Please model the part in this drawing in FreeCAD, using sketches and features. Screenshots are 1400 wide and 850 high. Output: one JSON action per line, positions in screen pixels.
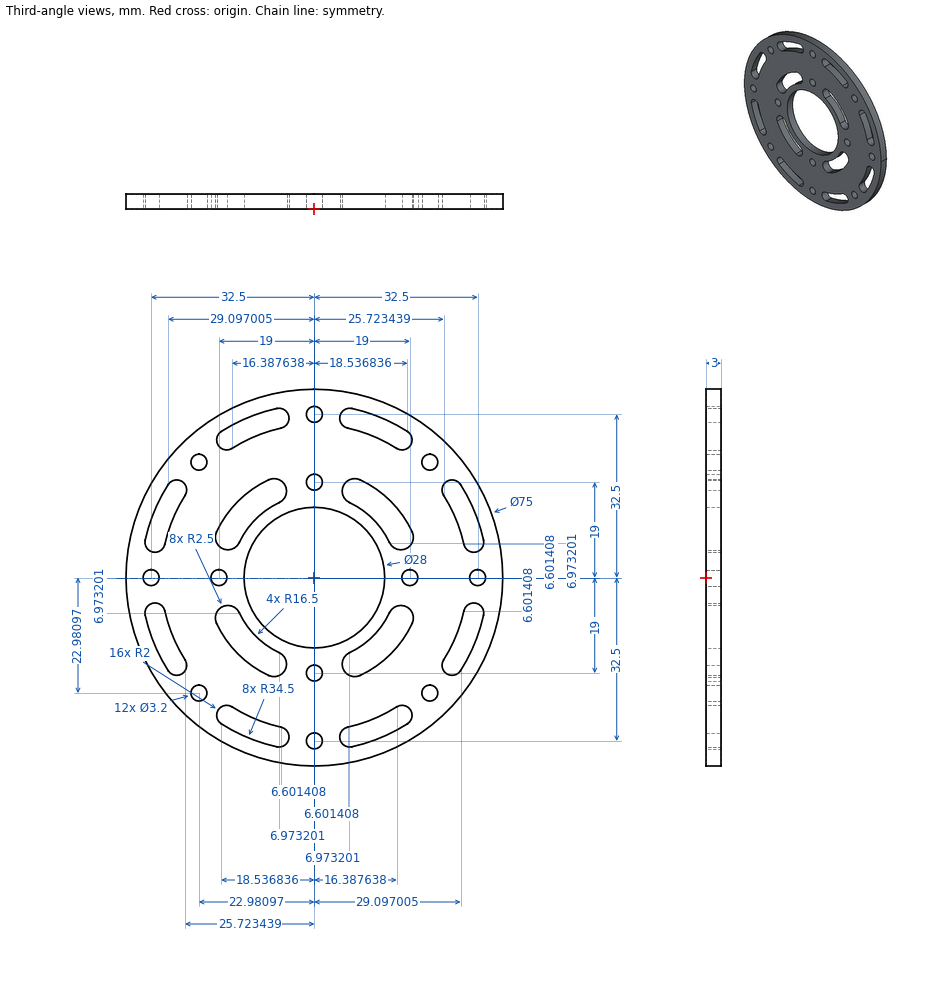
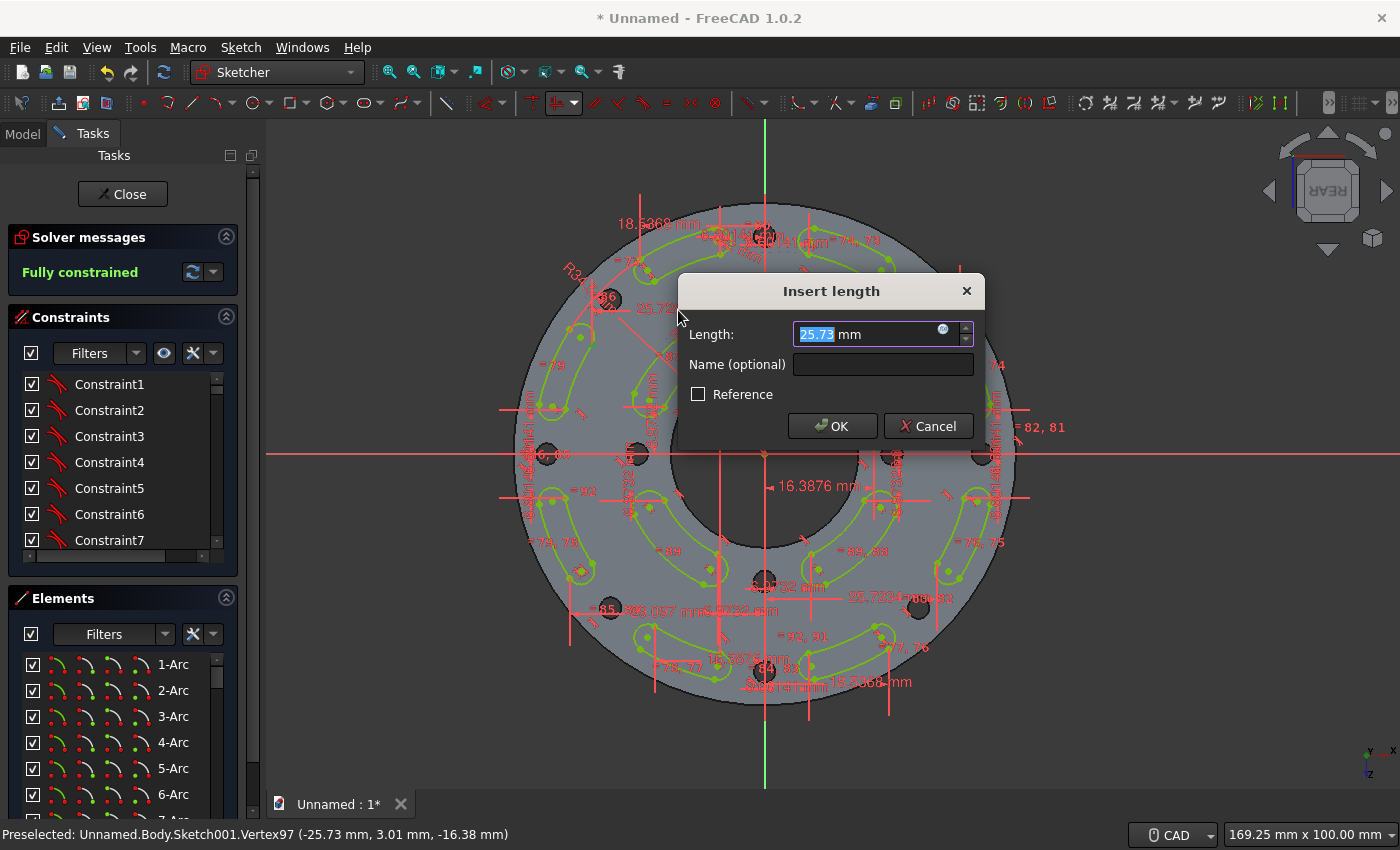
{"action": "type", "text": "25.723439"}
{"action": "key", "text": "Return"}
{"action": "key", "text": "Escape"}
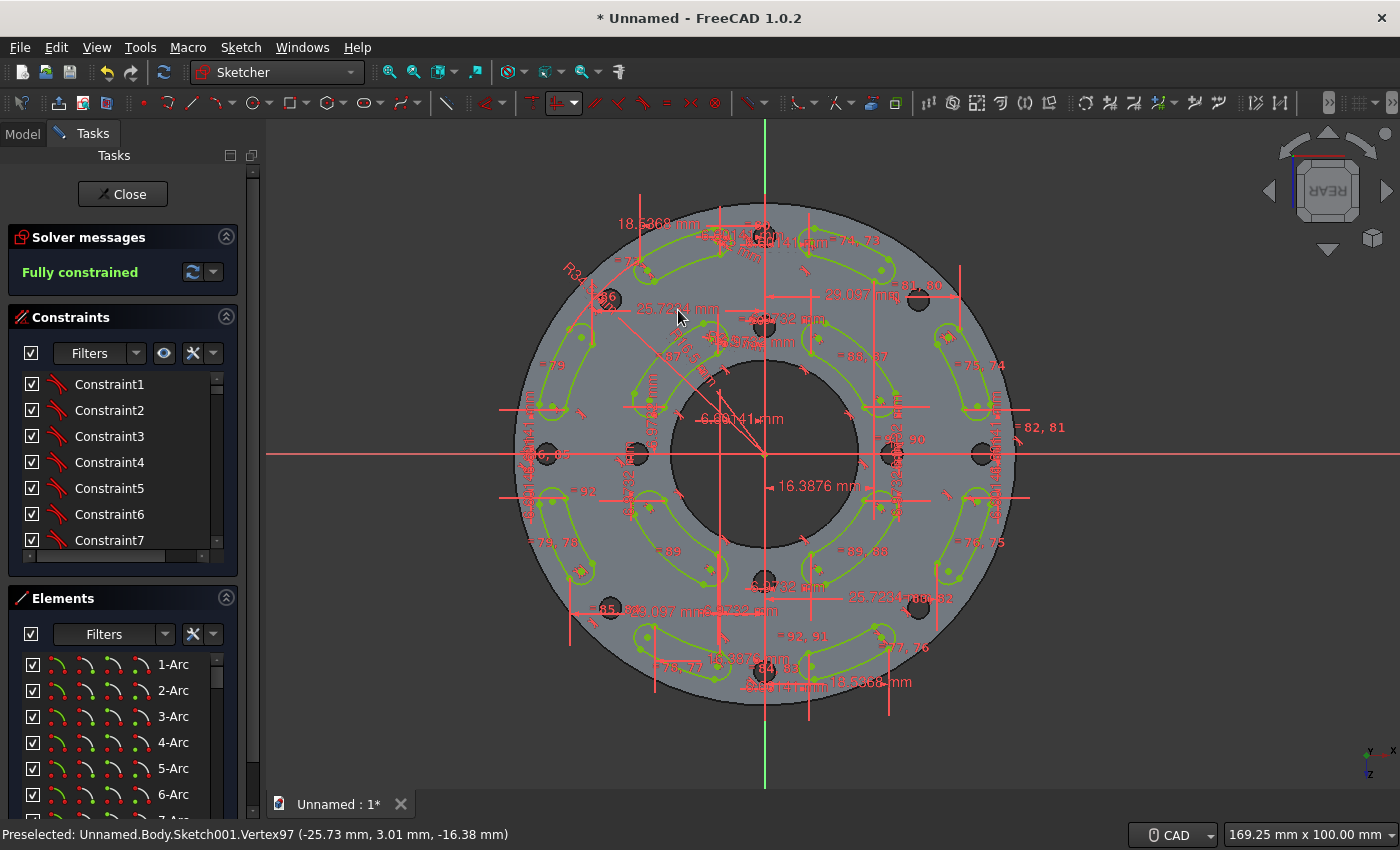
{"action": "left_click", "coordinate": [123, 194]}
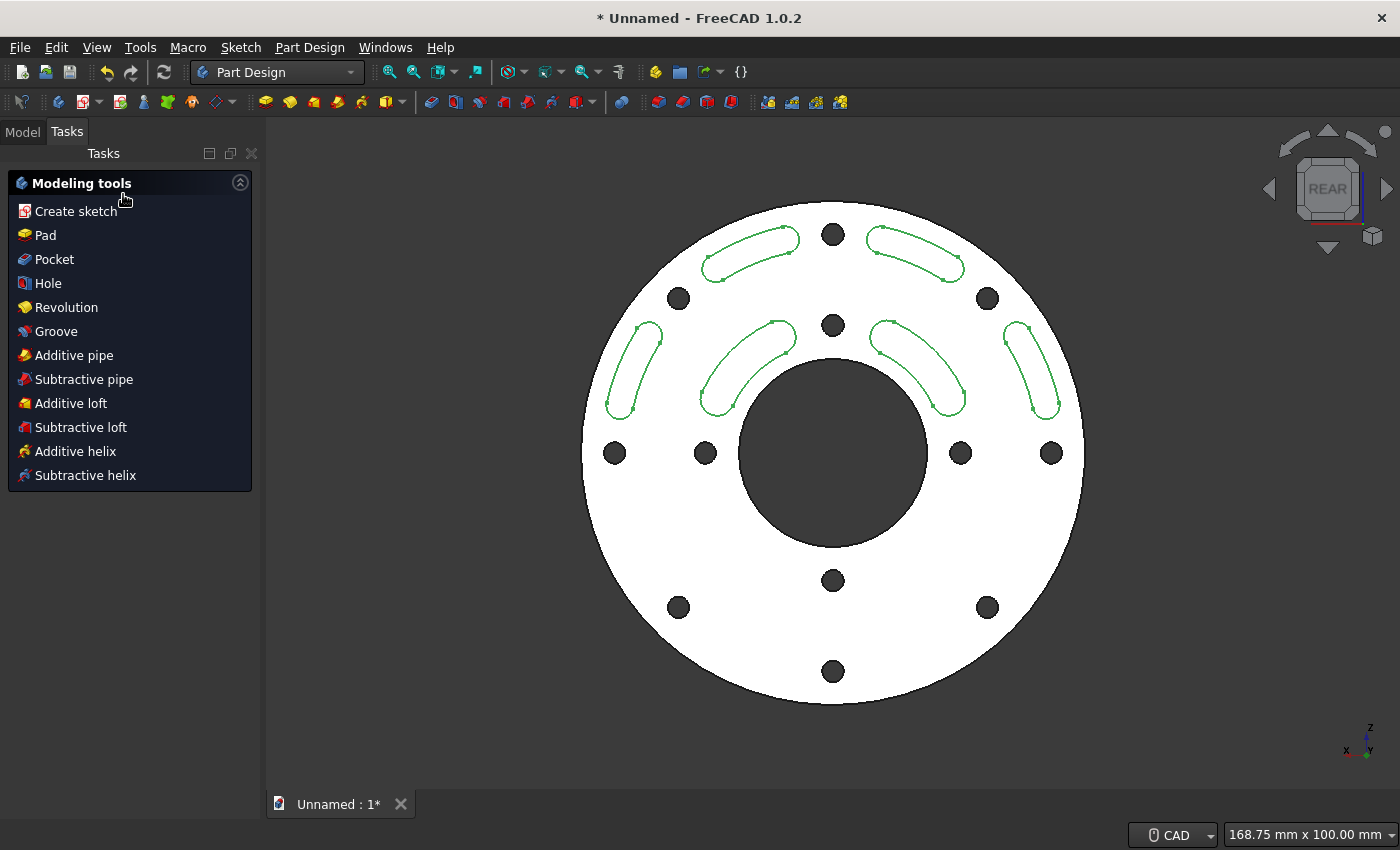
{"action": "left_click", "coordinate": [432, 102]}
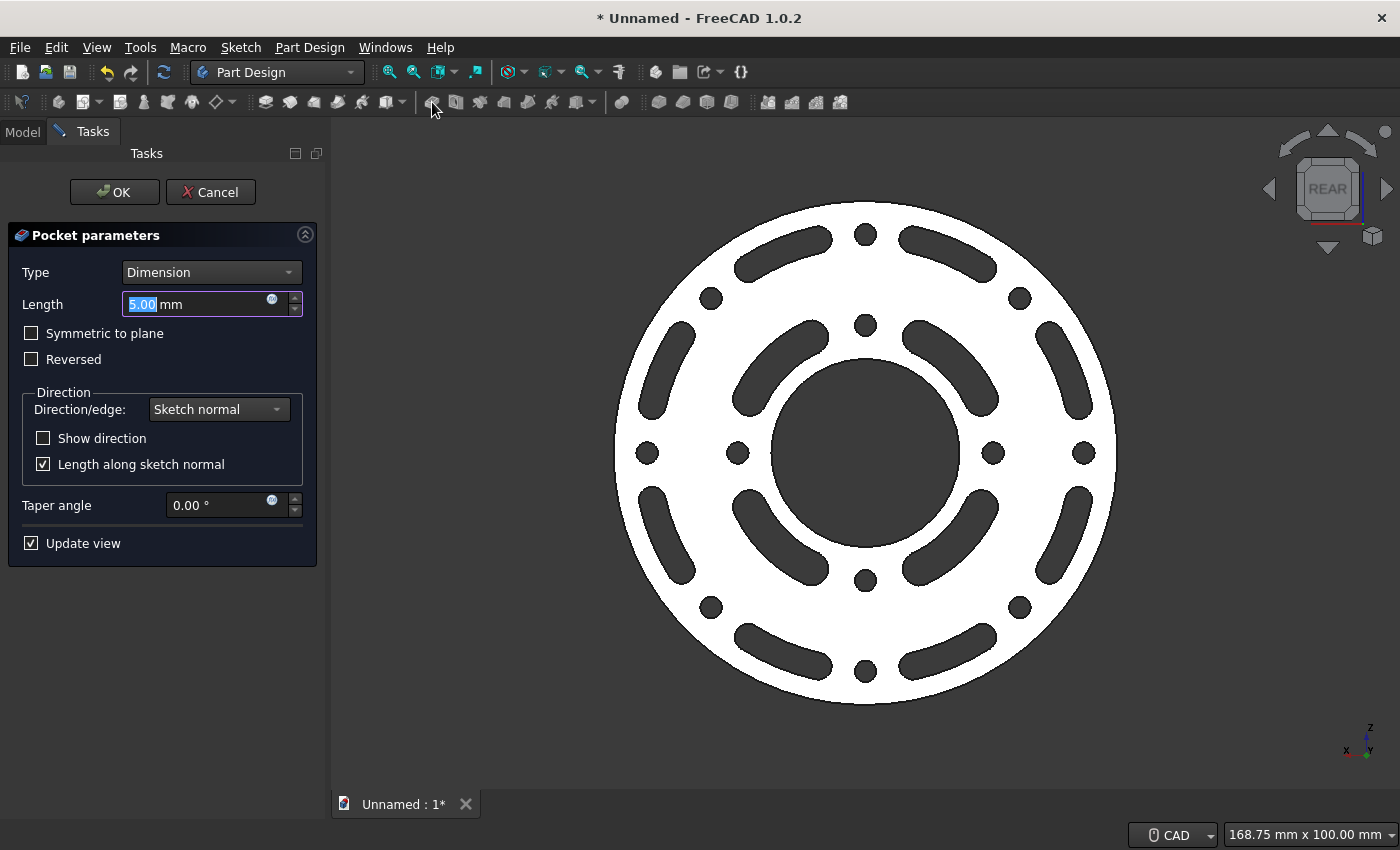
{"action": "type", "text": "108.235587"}
{"action": "key", "text": "Tab"}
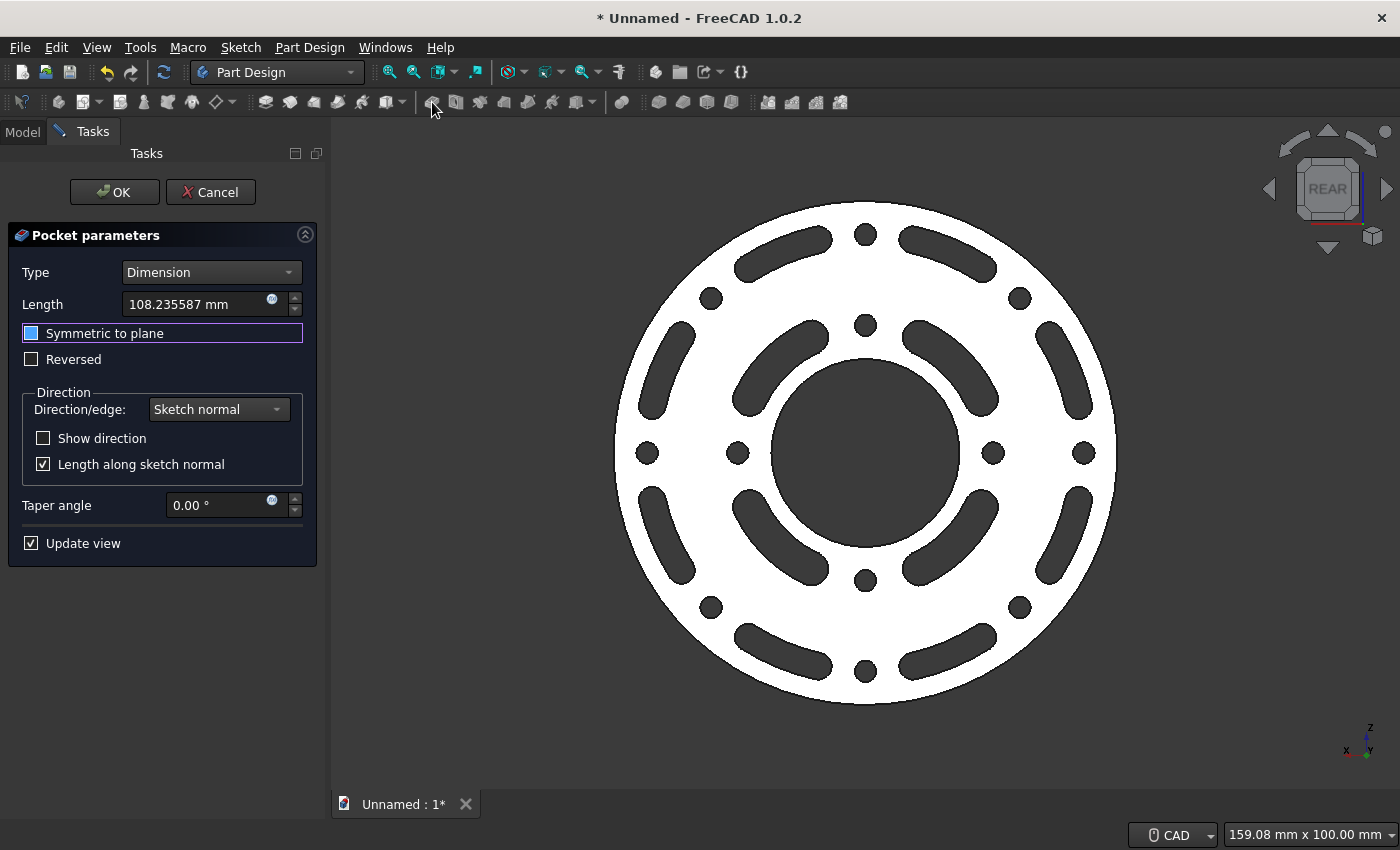
{"action": "left_click", "coordinate": [30, 333]}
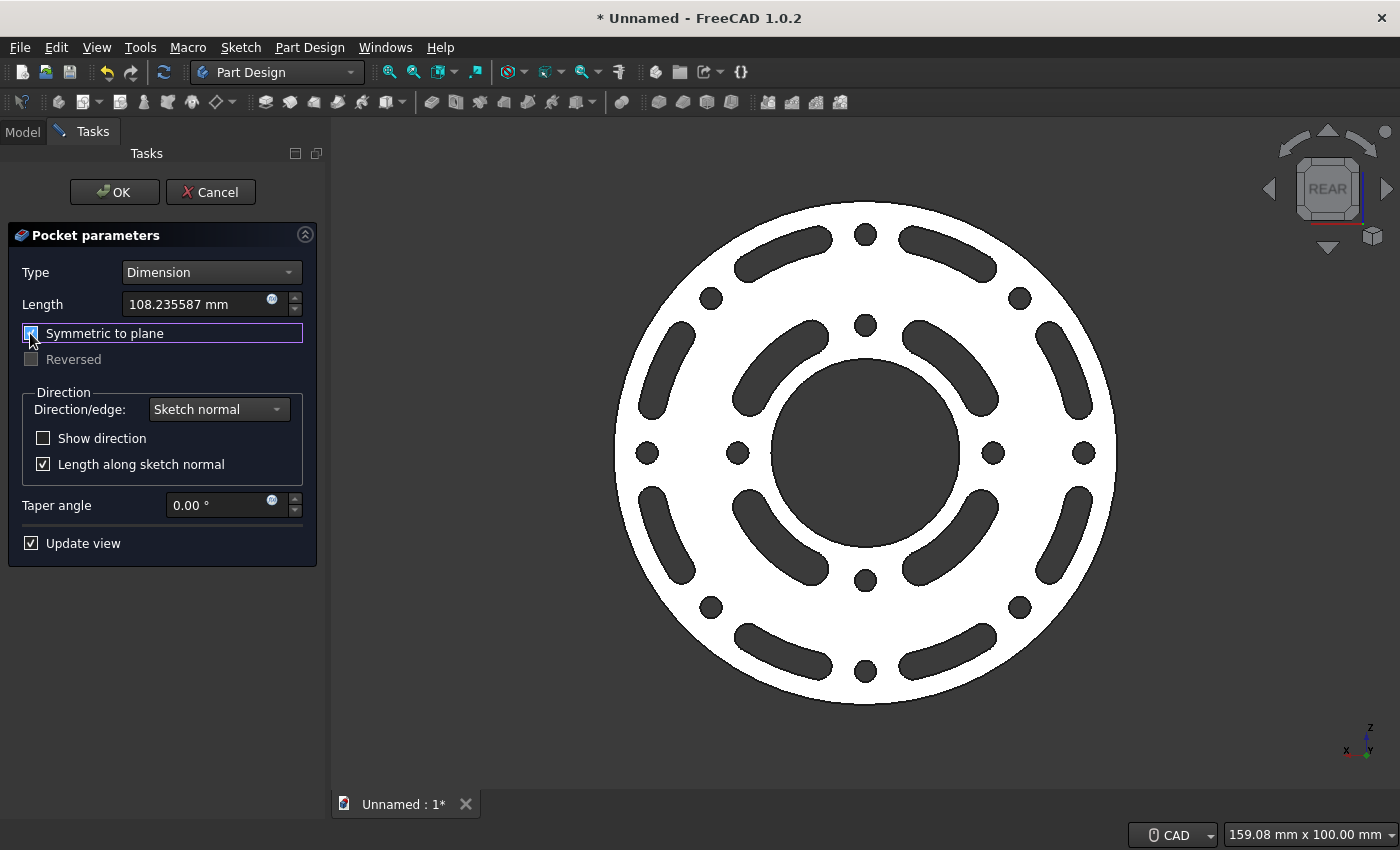
{"action": "left_click", "coordinate": [115, 192]}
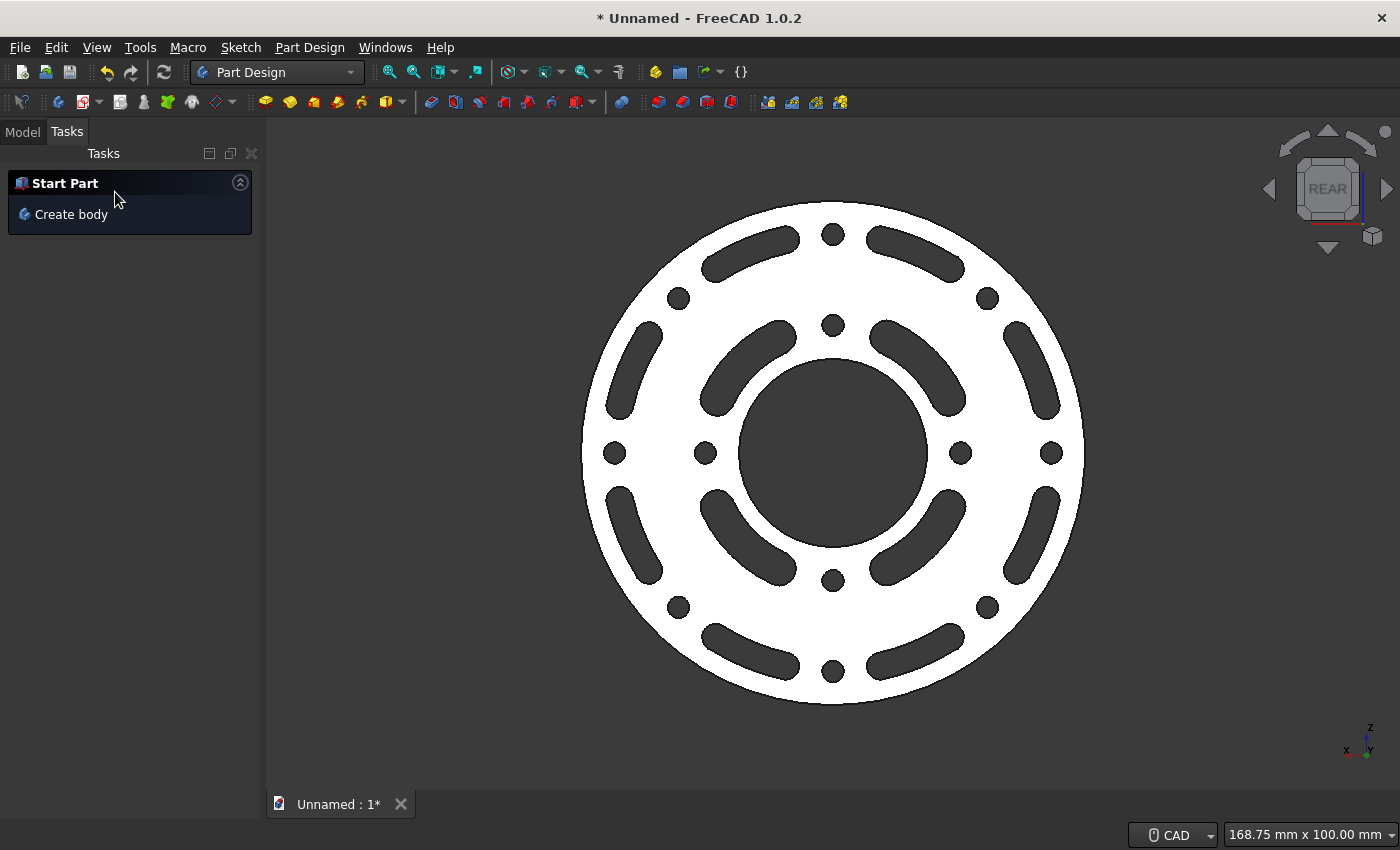
{"action": "key", "text": "0"}